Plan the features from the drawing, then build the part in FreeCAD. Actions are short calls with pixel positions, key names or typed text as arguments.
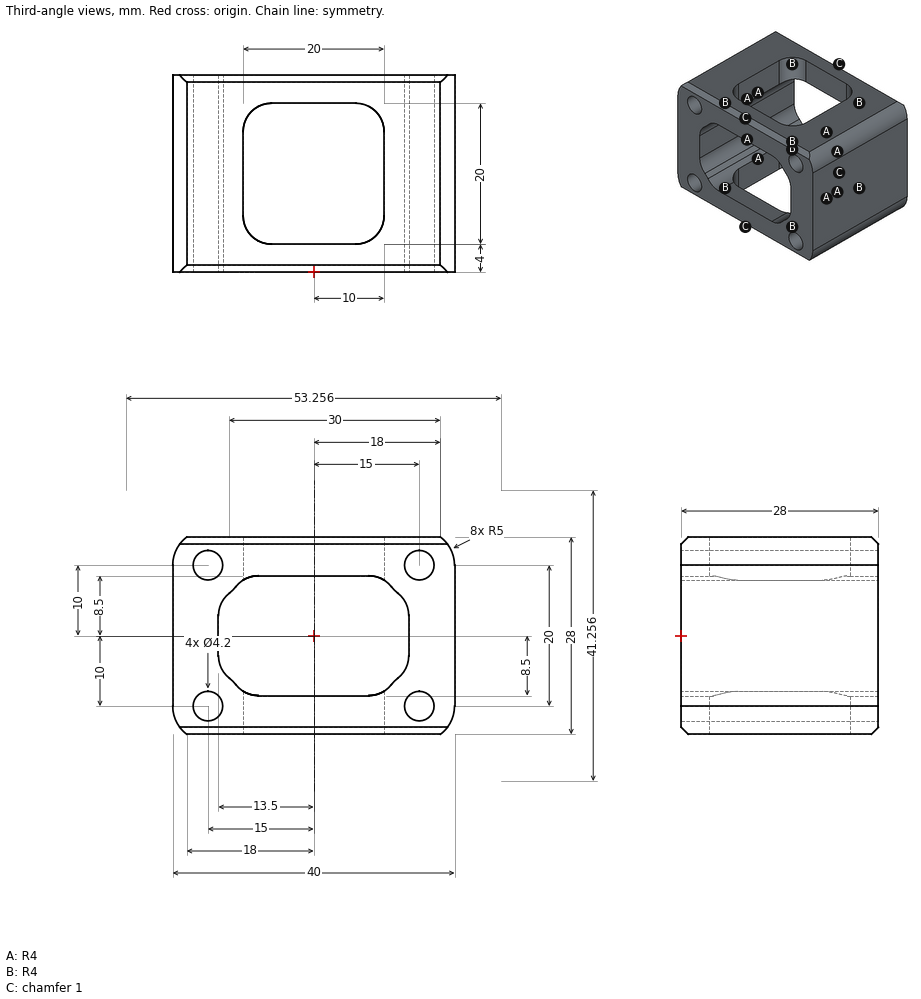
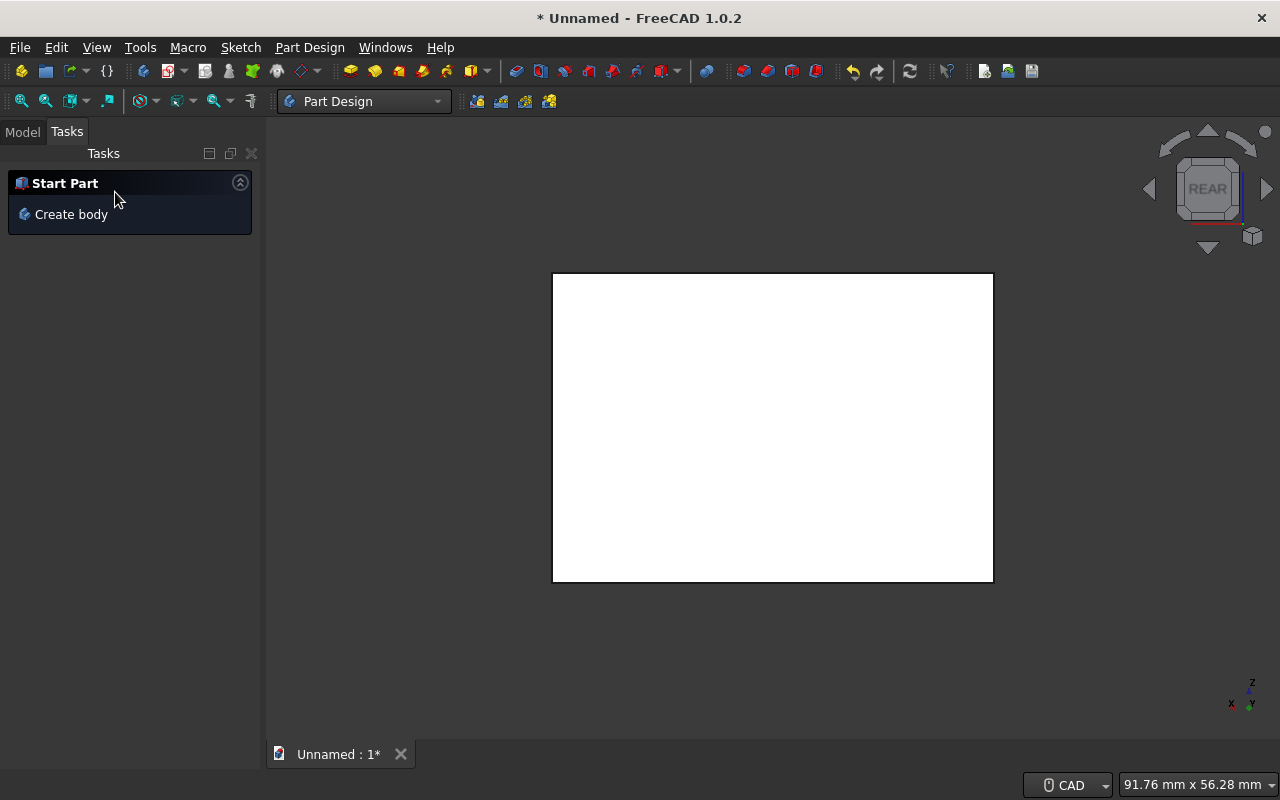
click(710, 427)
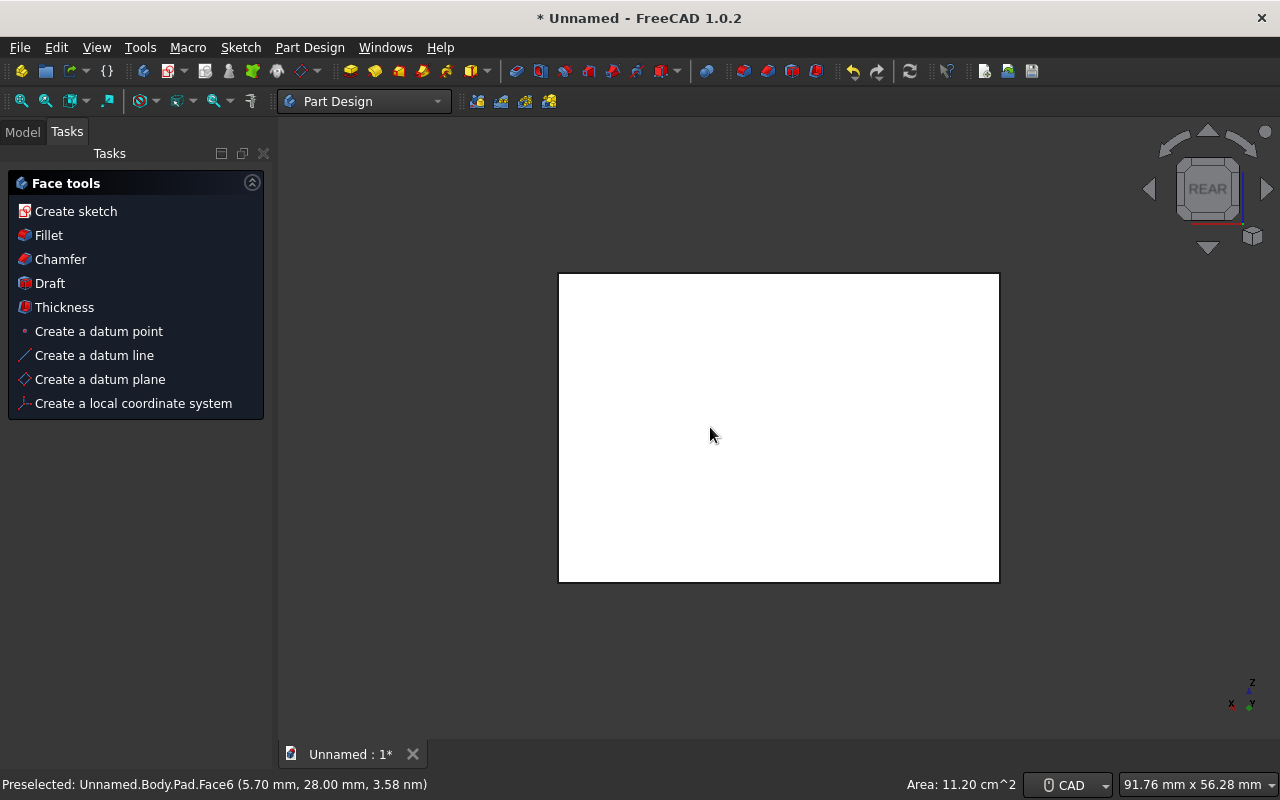
click(168, 72)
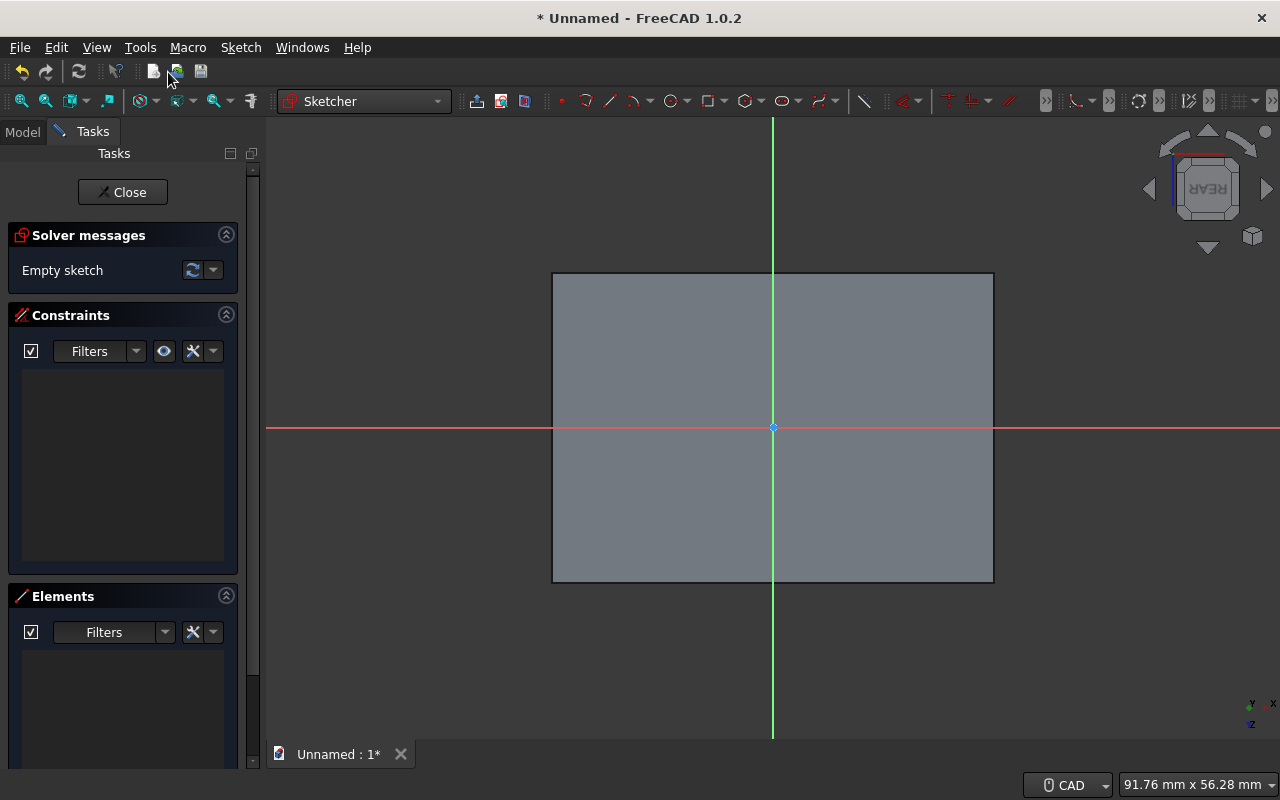
scroll(912, 428, up, 2)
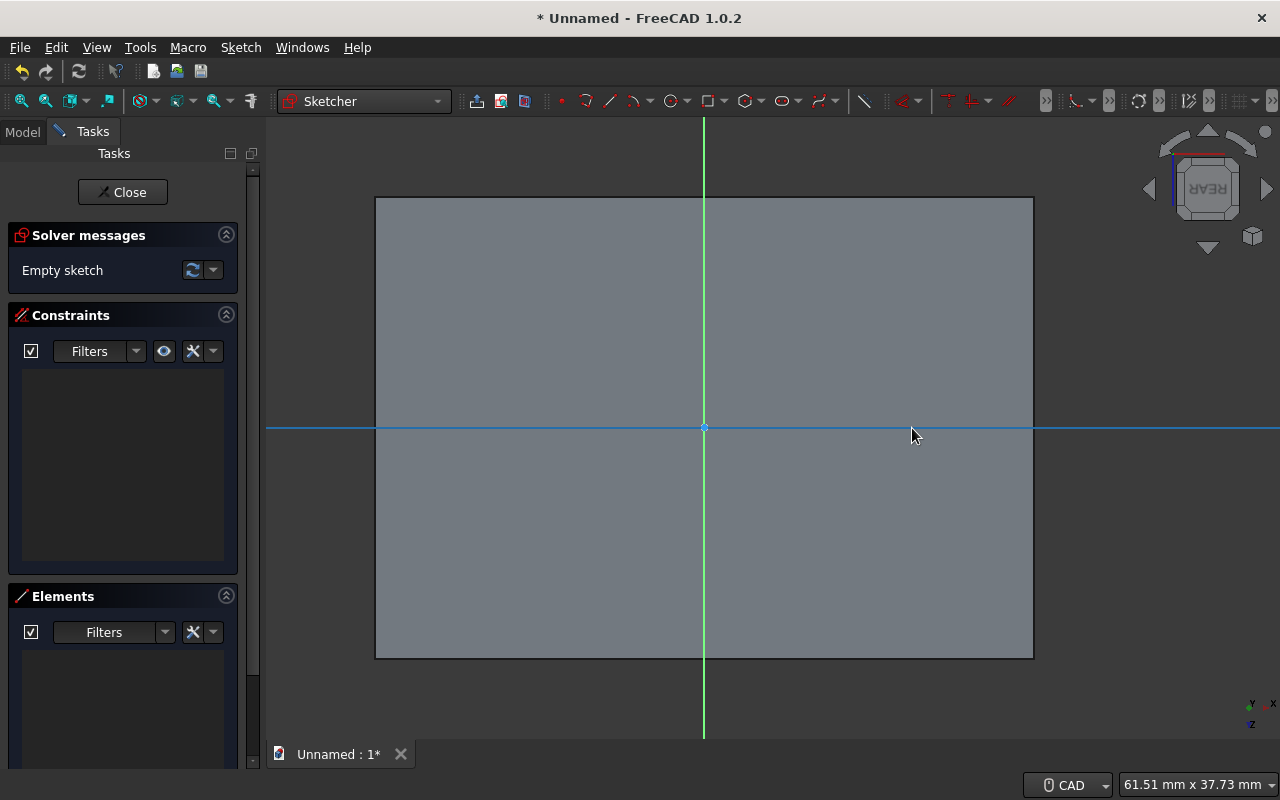
click(672, 102)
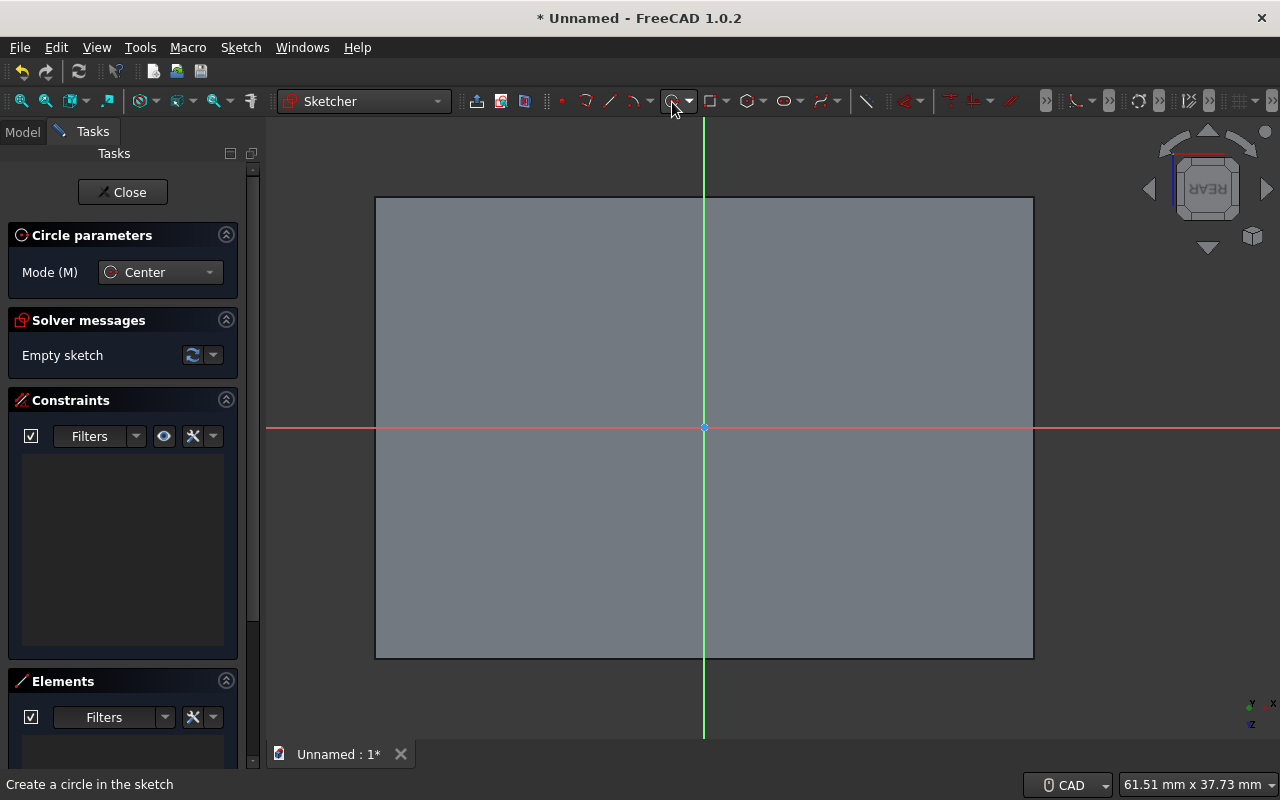
click(457, 263)
click(482, 238)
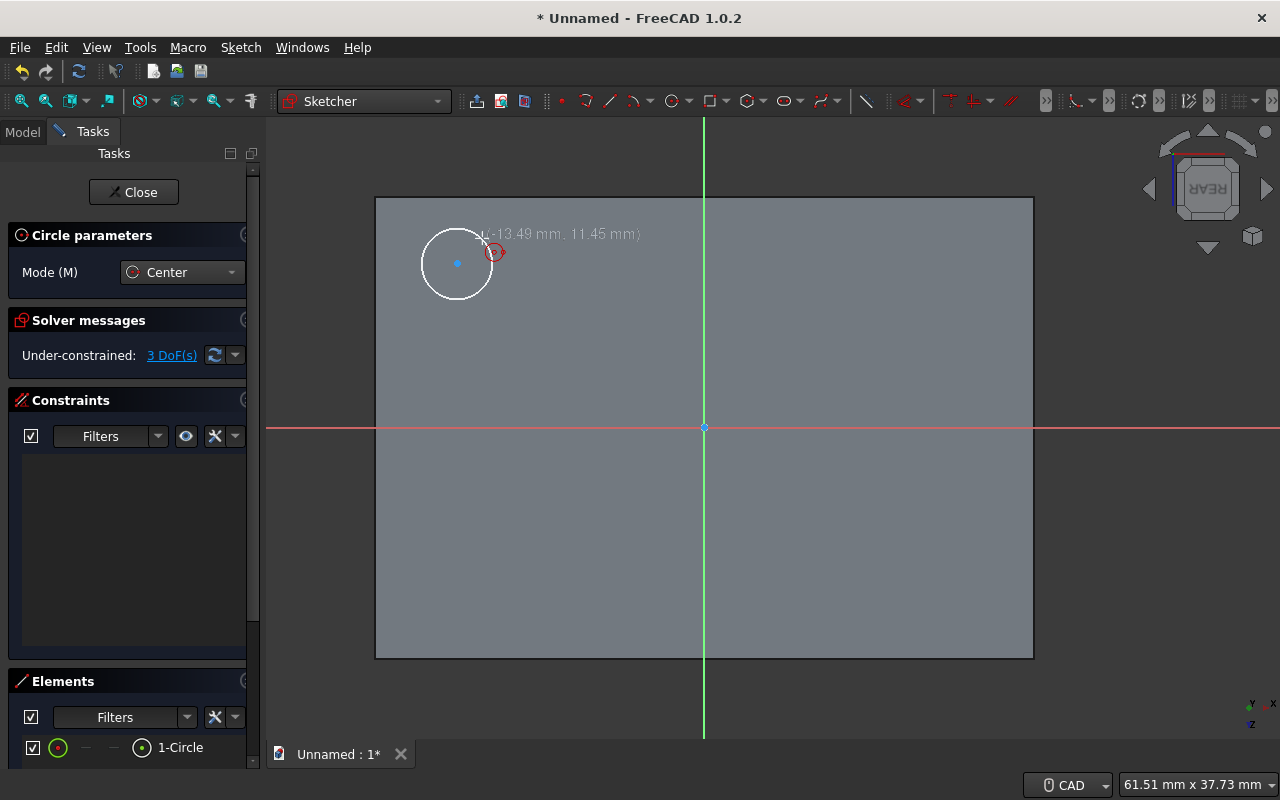
click(457, 593)
click(482, 568)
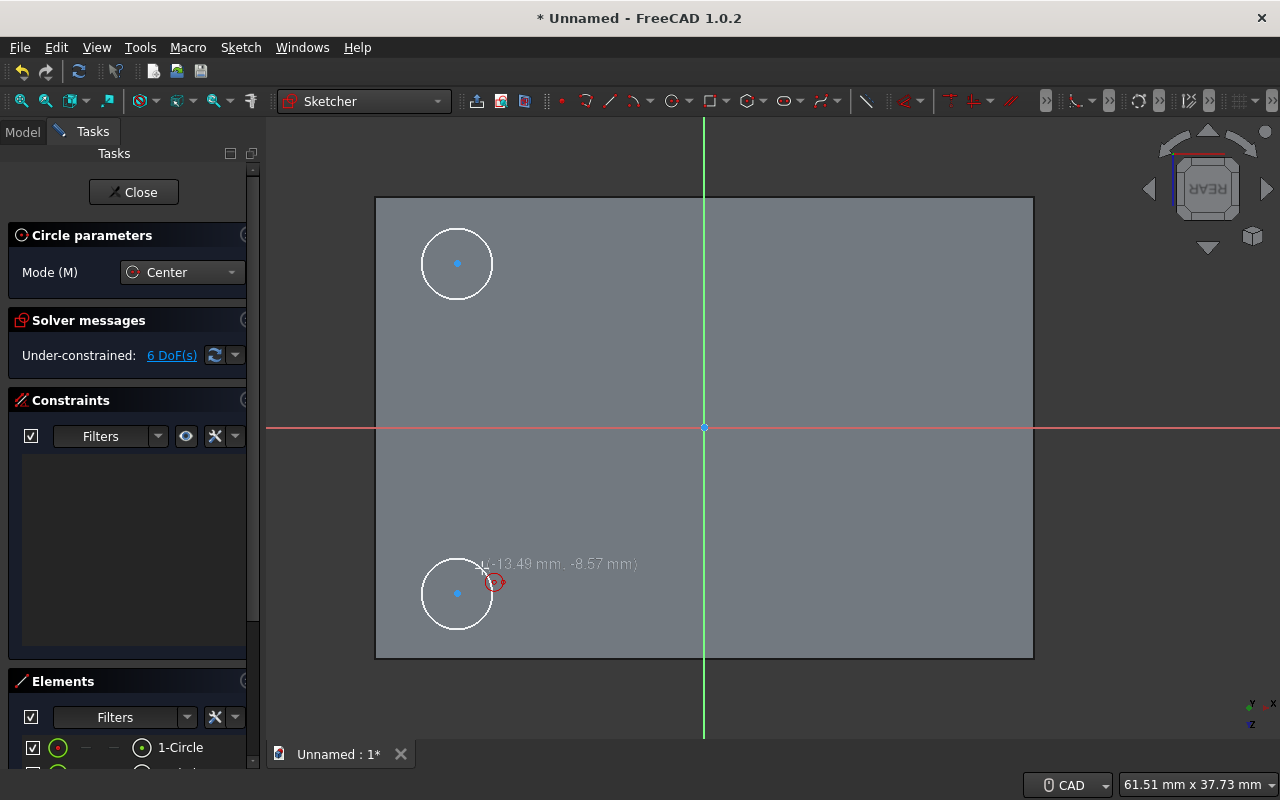
click(952, 593)
click(976, 568)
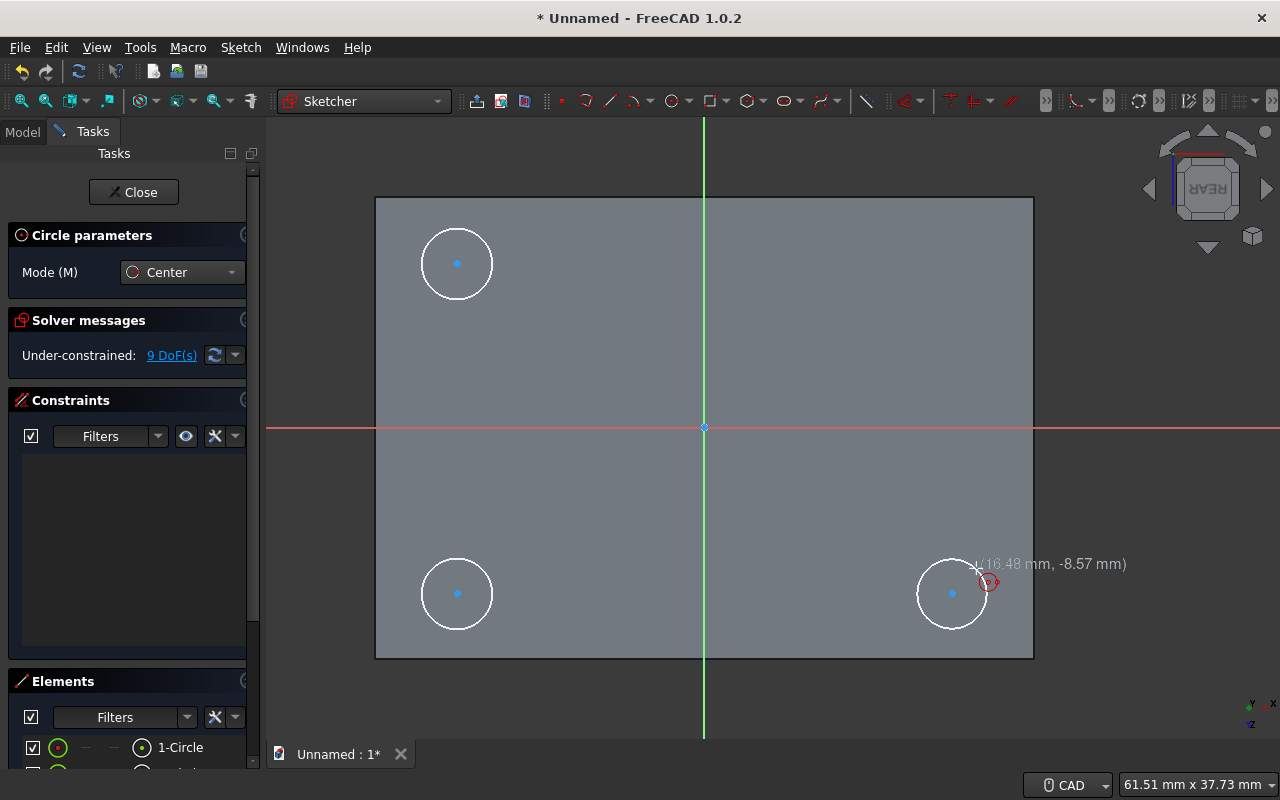
click(952, 263)
click(976, 238)
key(Escape)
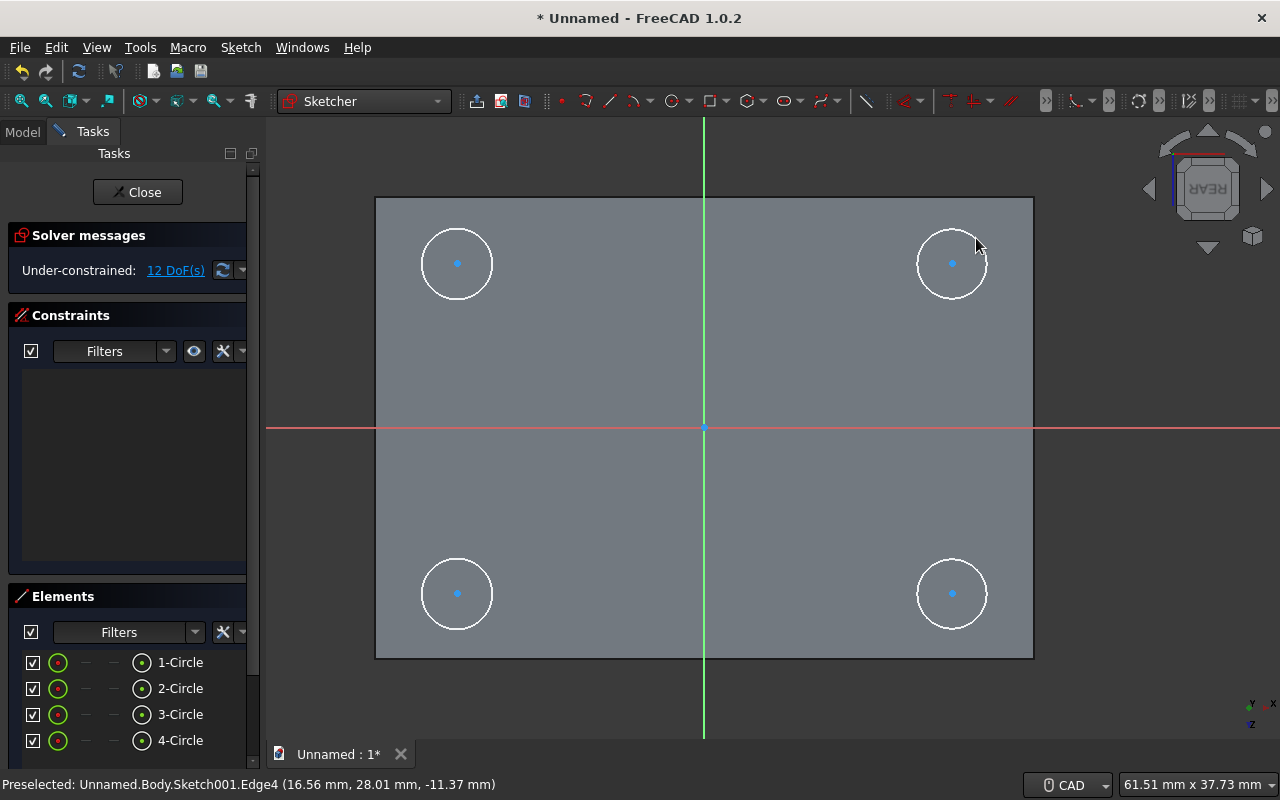
click(482, 239)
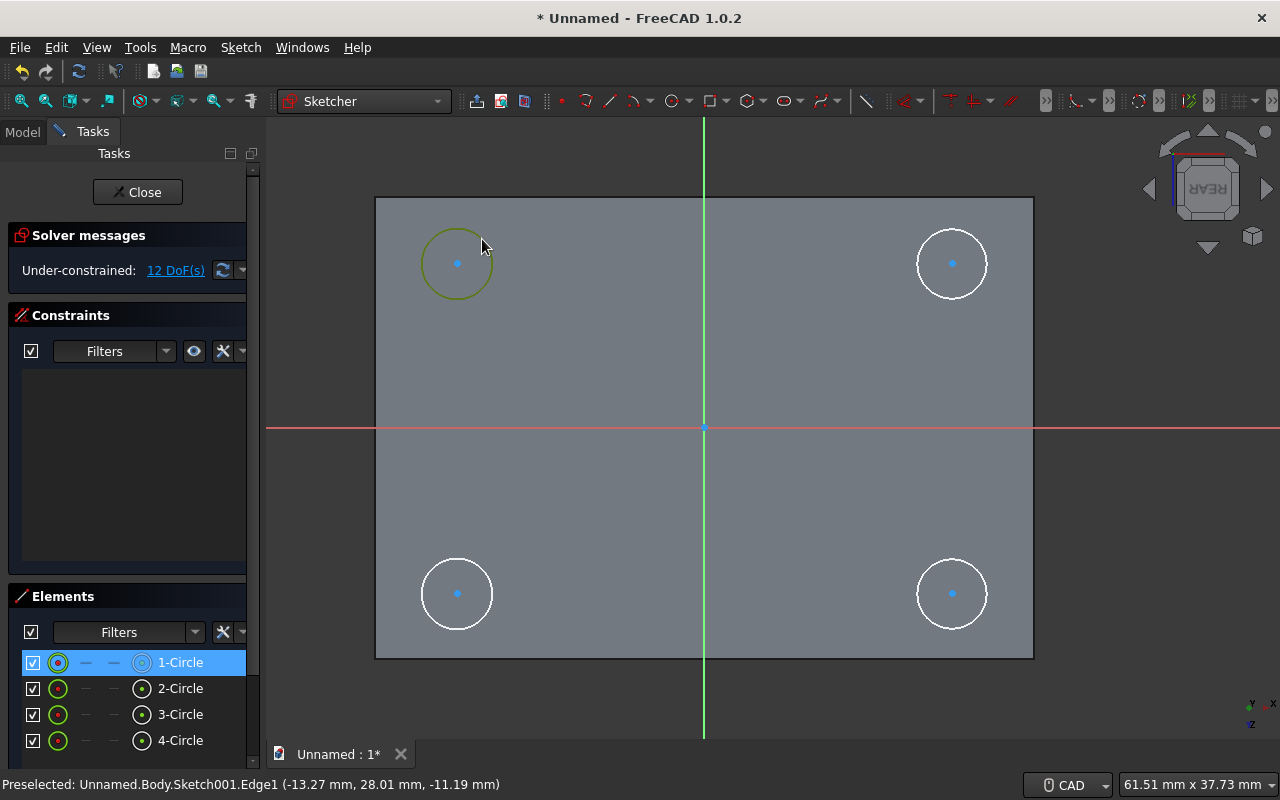
click(482, 569)